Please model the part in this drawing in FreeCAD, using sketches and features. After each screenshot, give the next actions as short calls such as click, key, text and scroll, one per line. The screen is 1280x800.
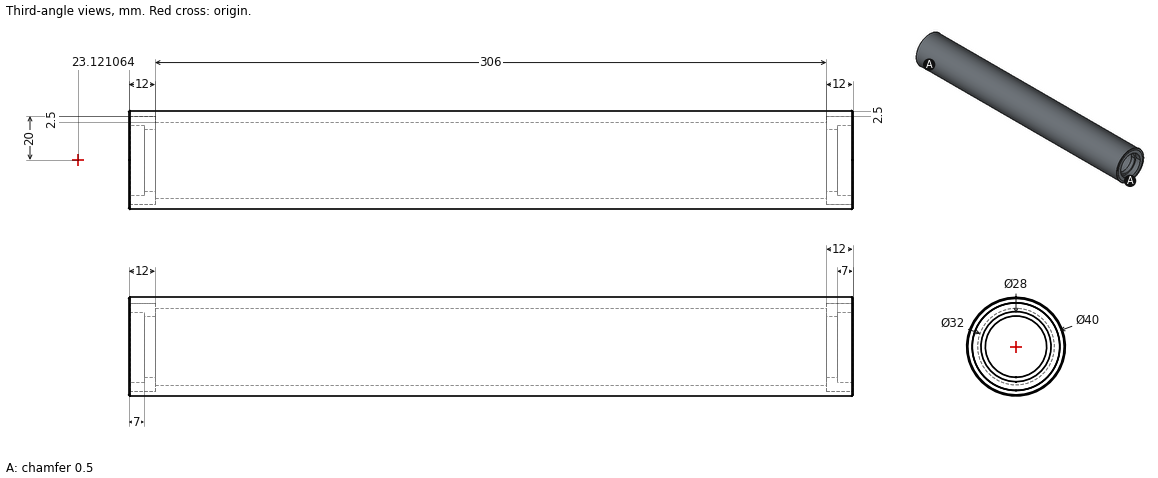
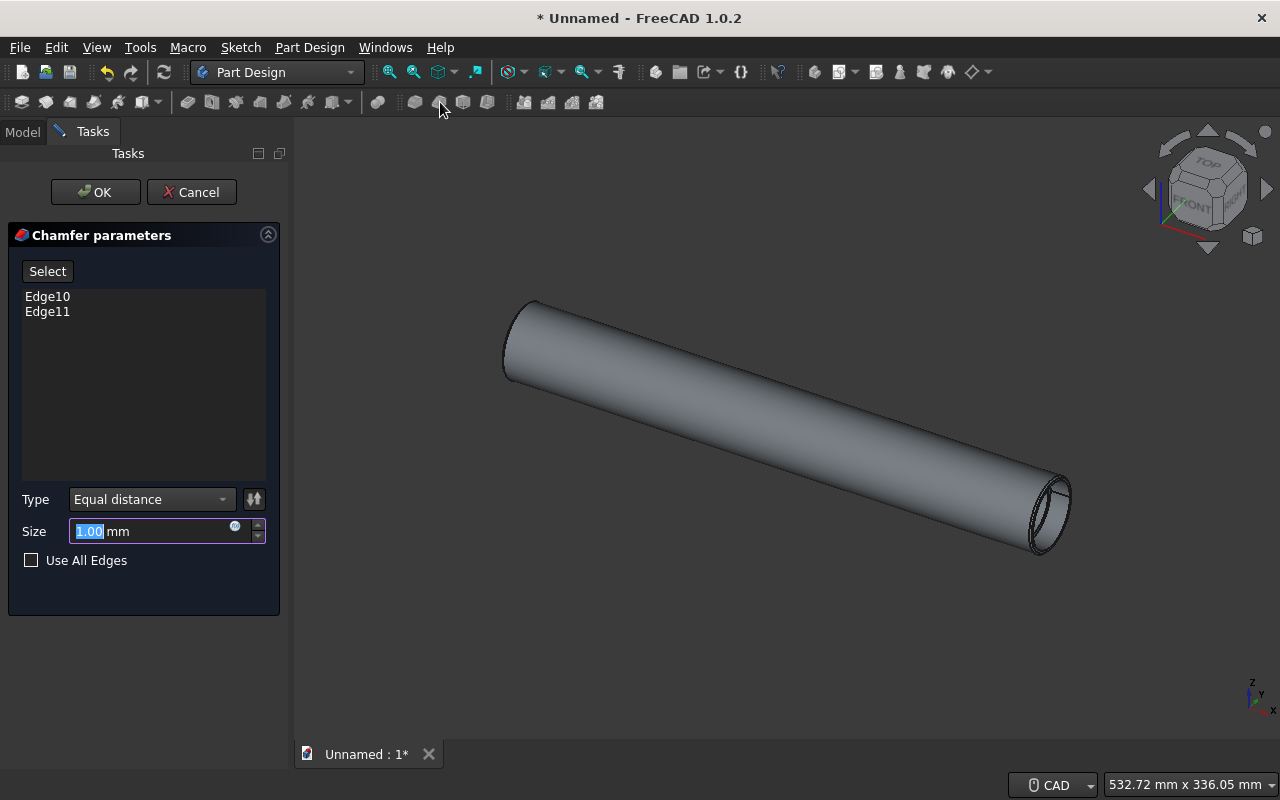
text(0.5)
key(Tab)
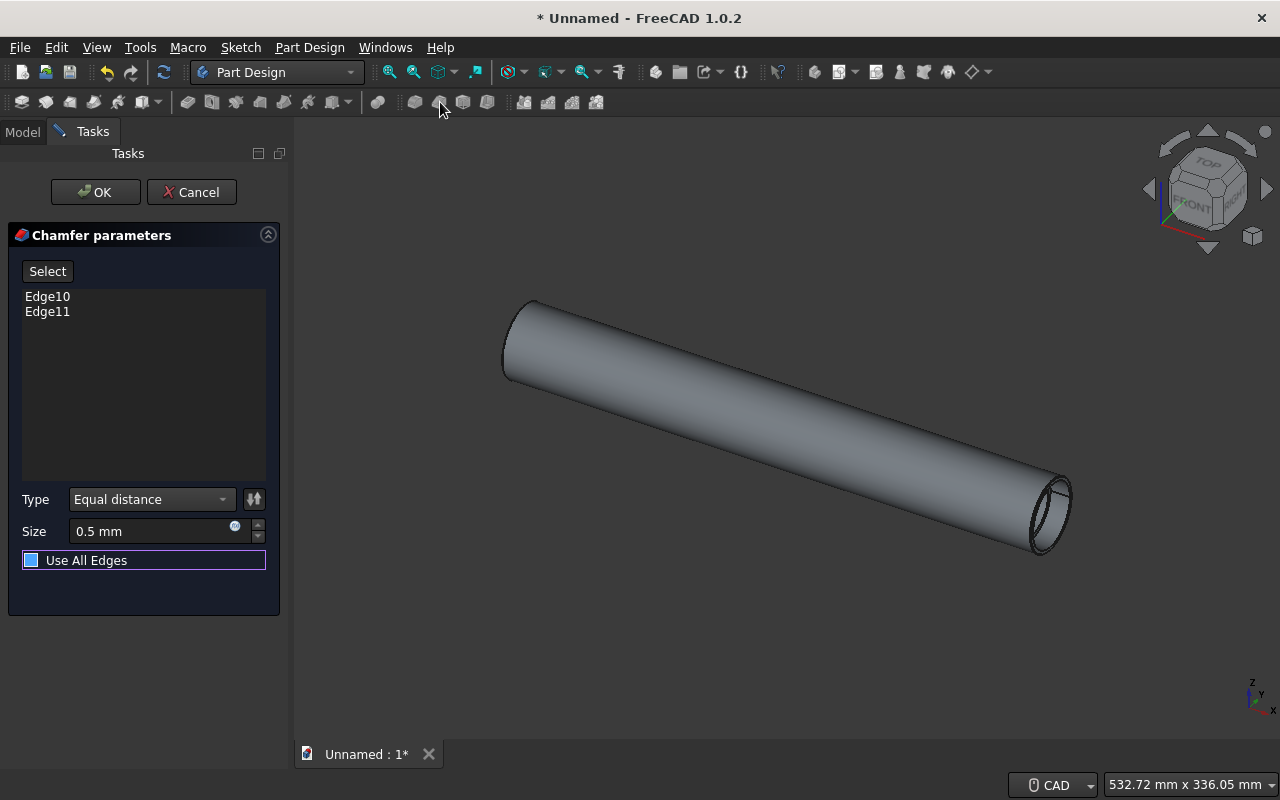
click(96, 192)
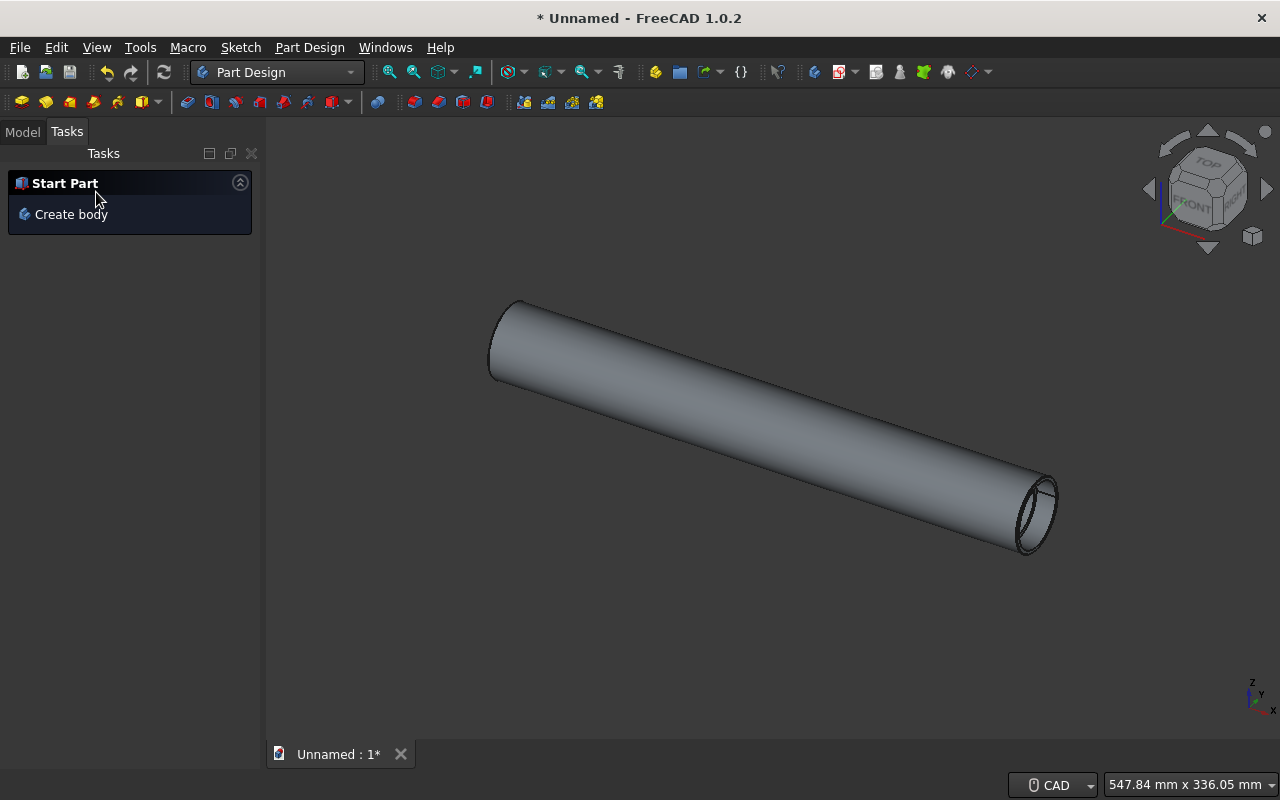
click(816, 72)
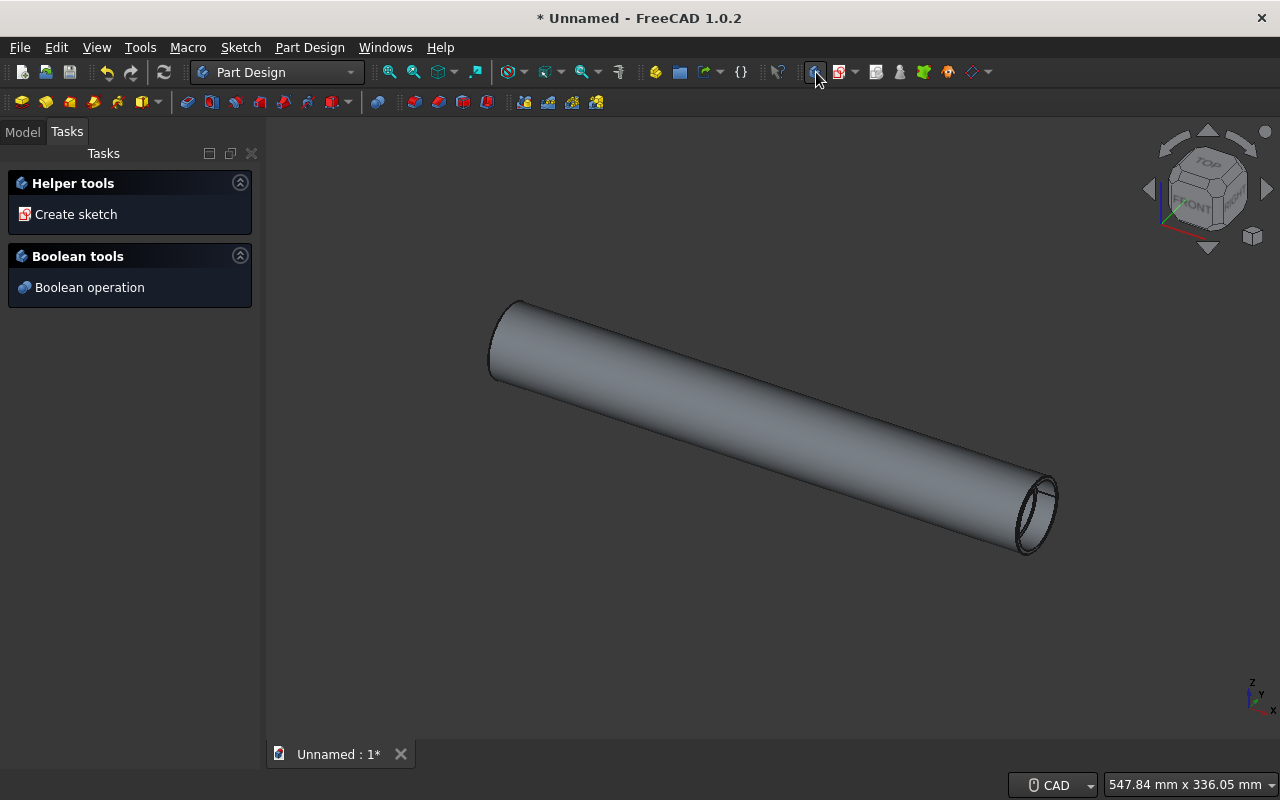
click(23, 131)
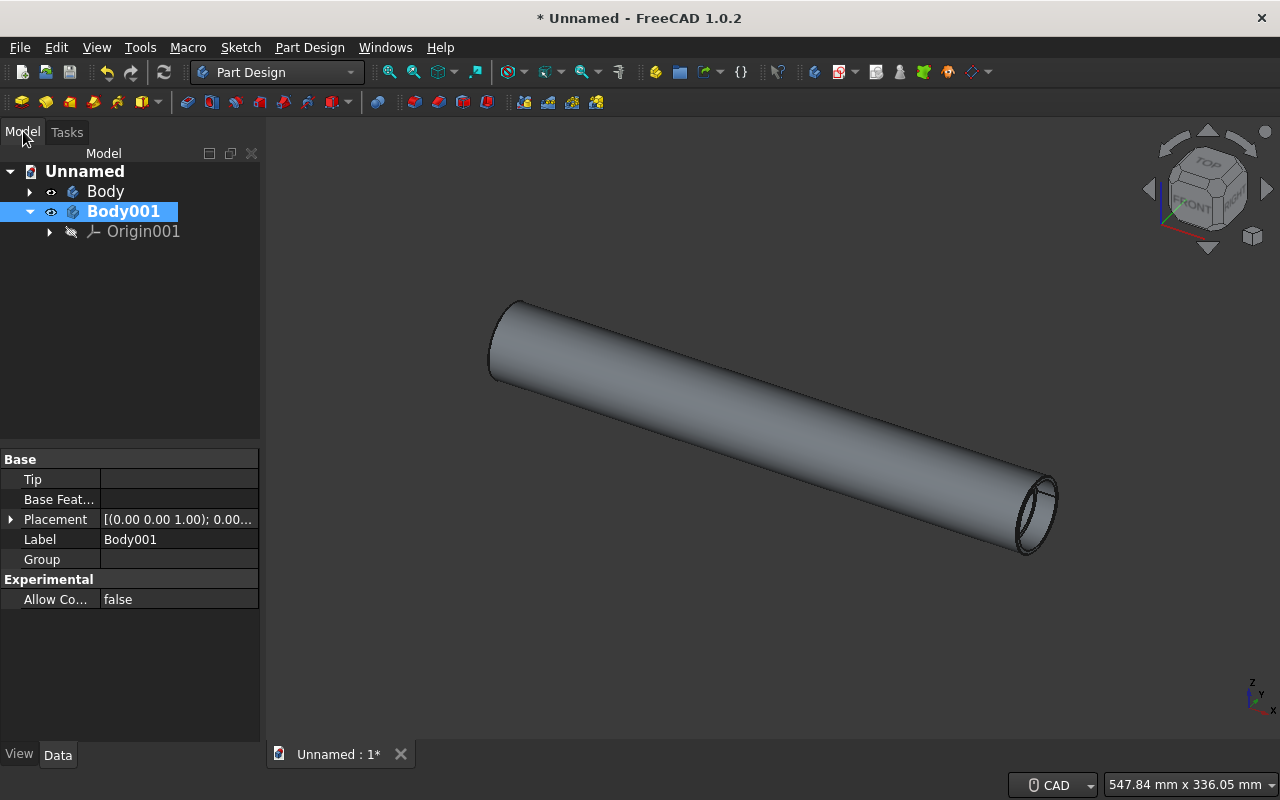
click(50, 232)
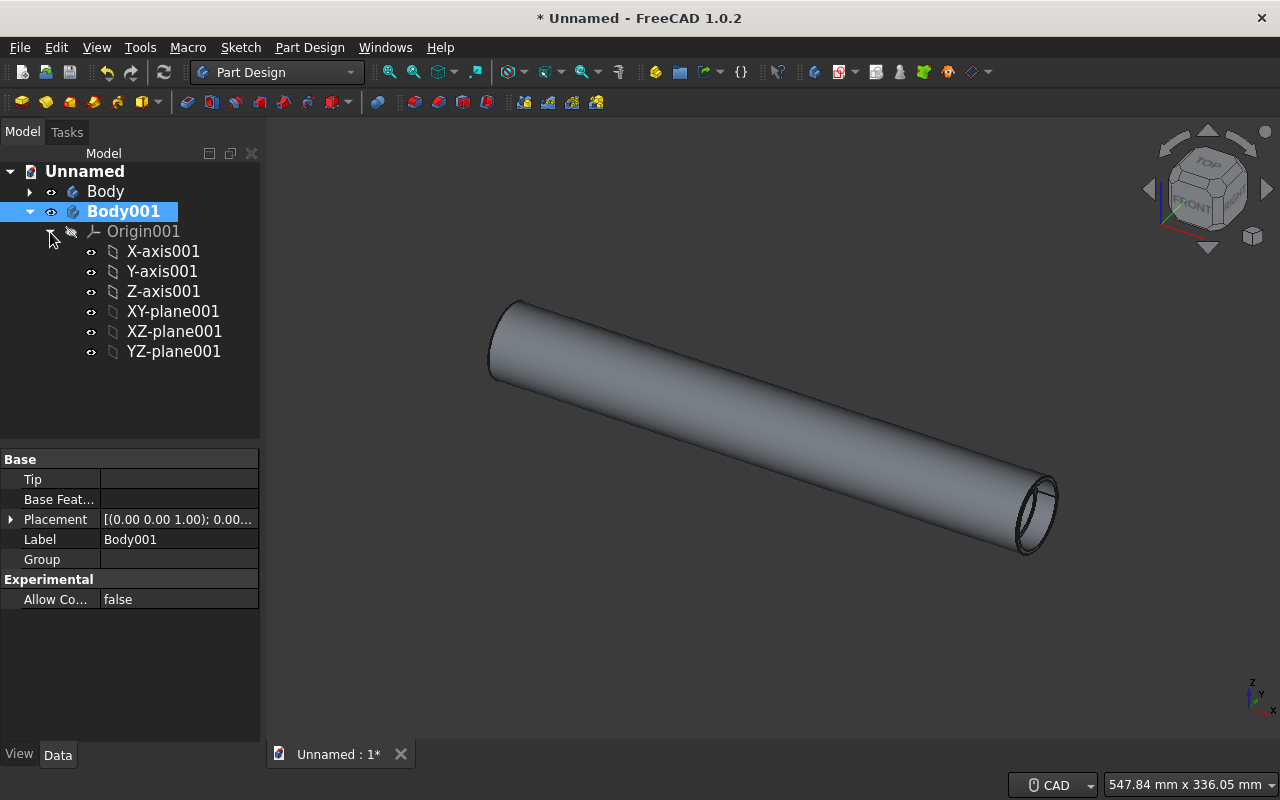
click(136, 352)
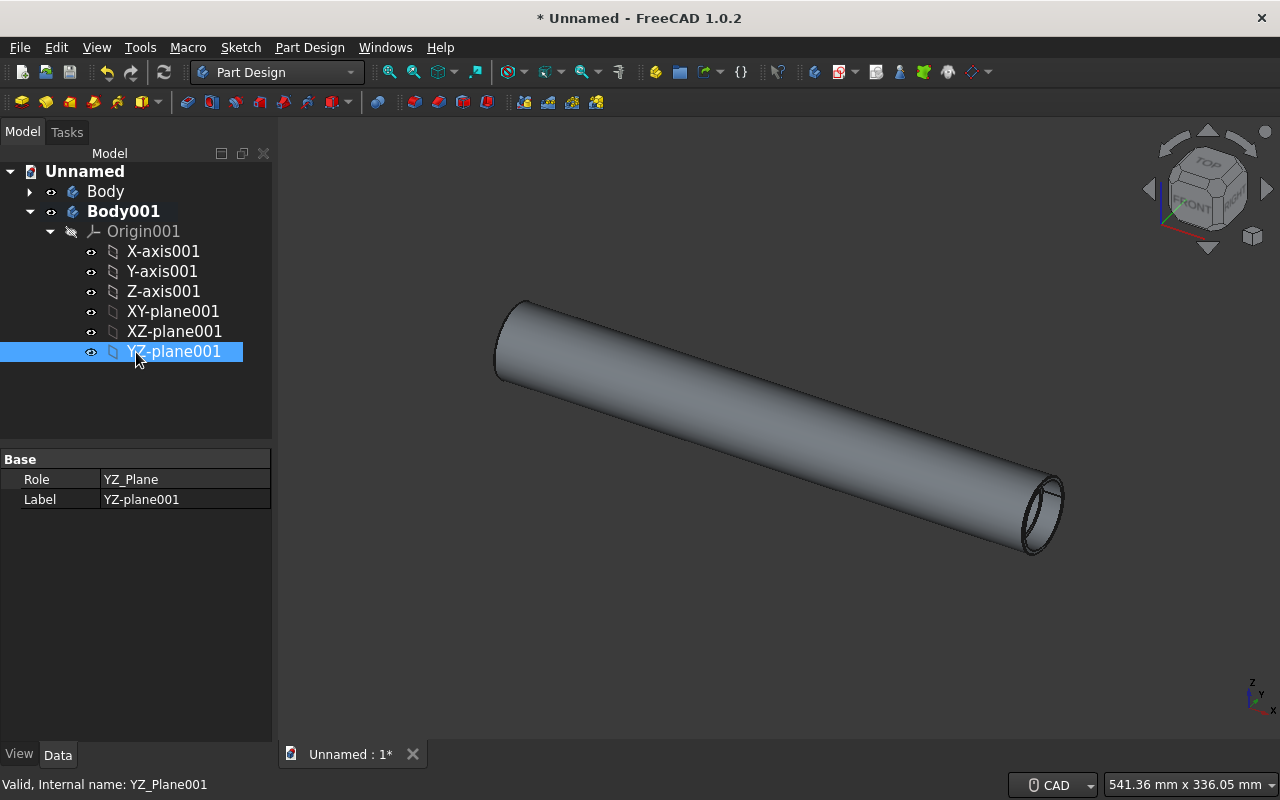
click(972, 72)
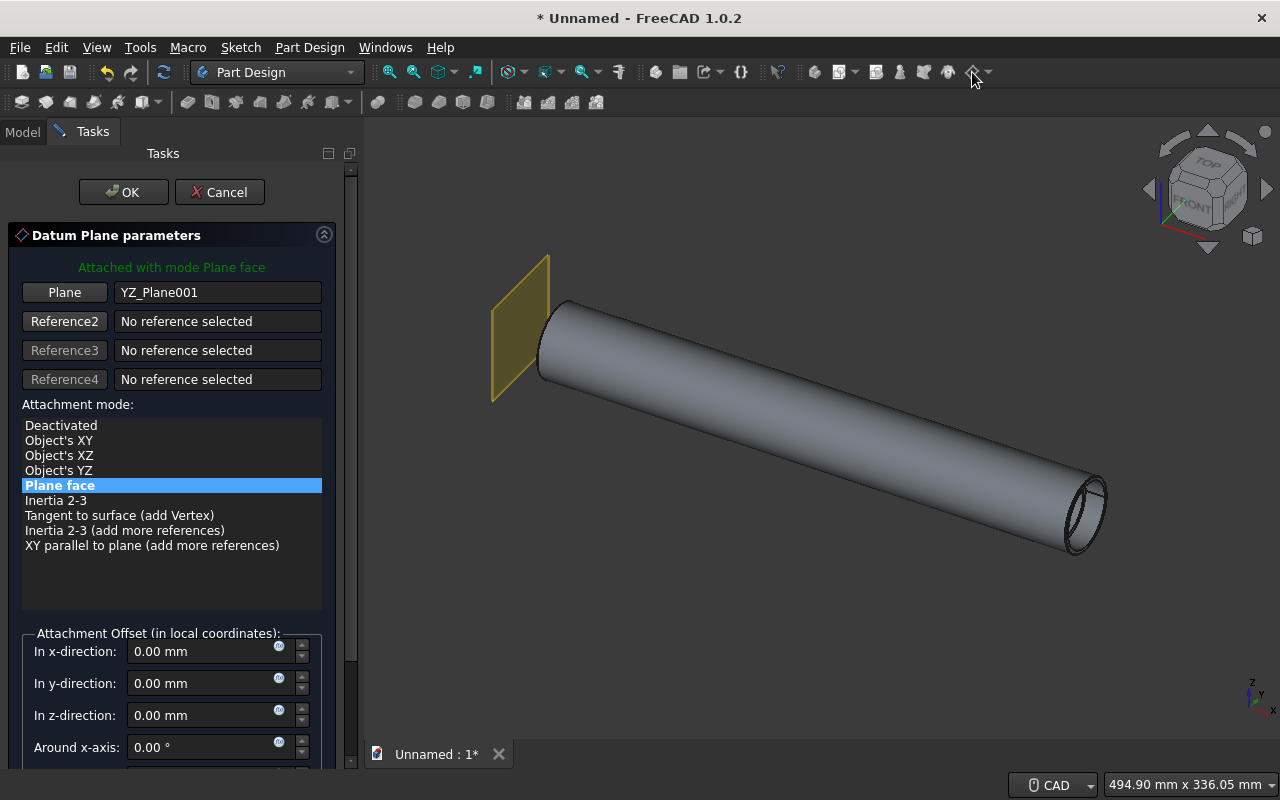
triple_click(210, 715)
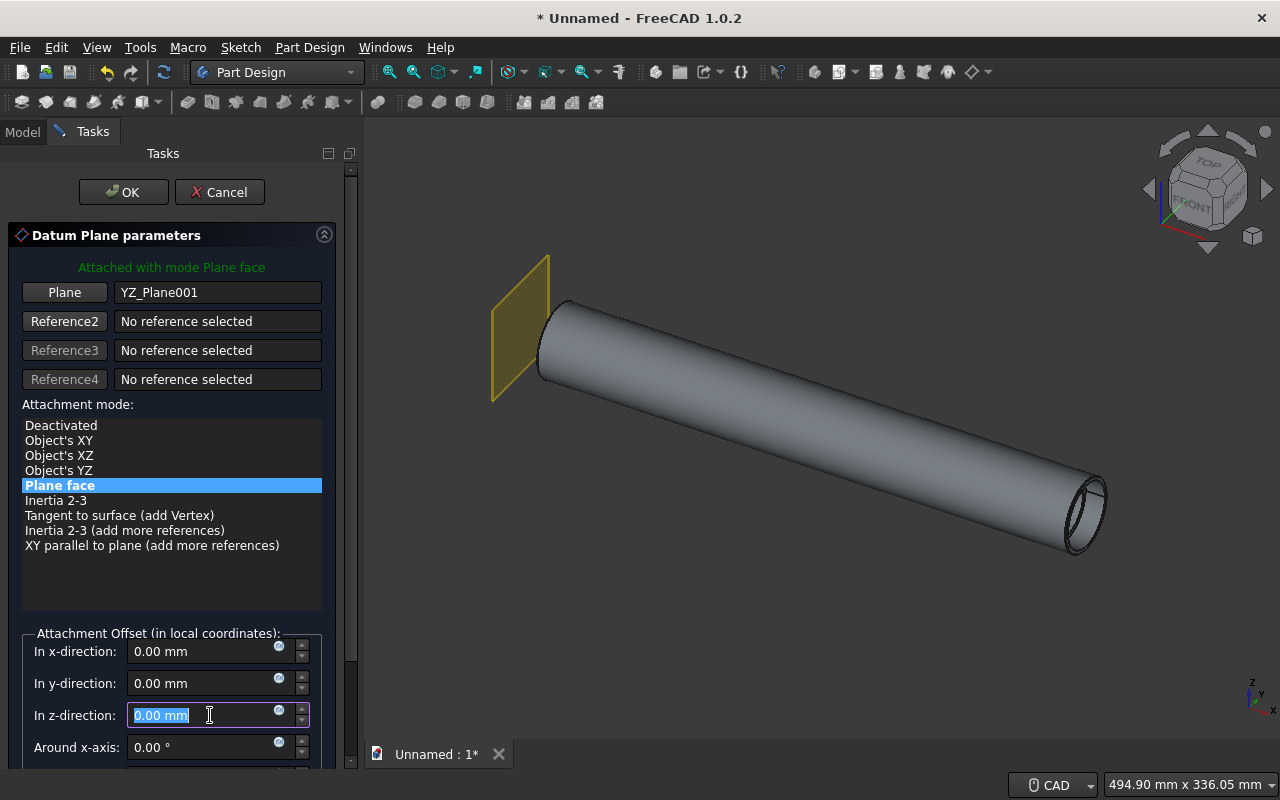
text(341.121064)
key(Tab)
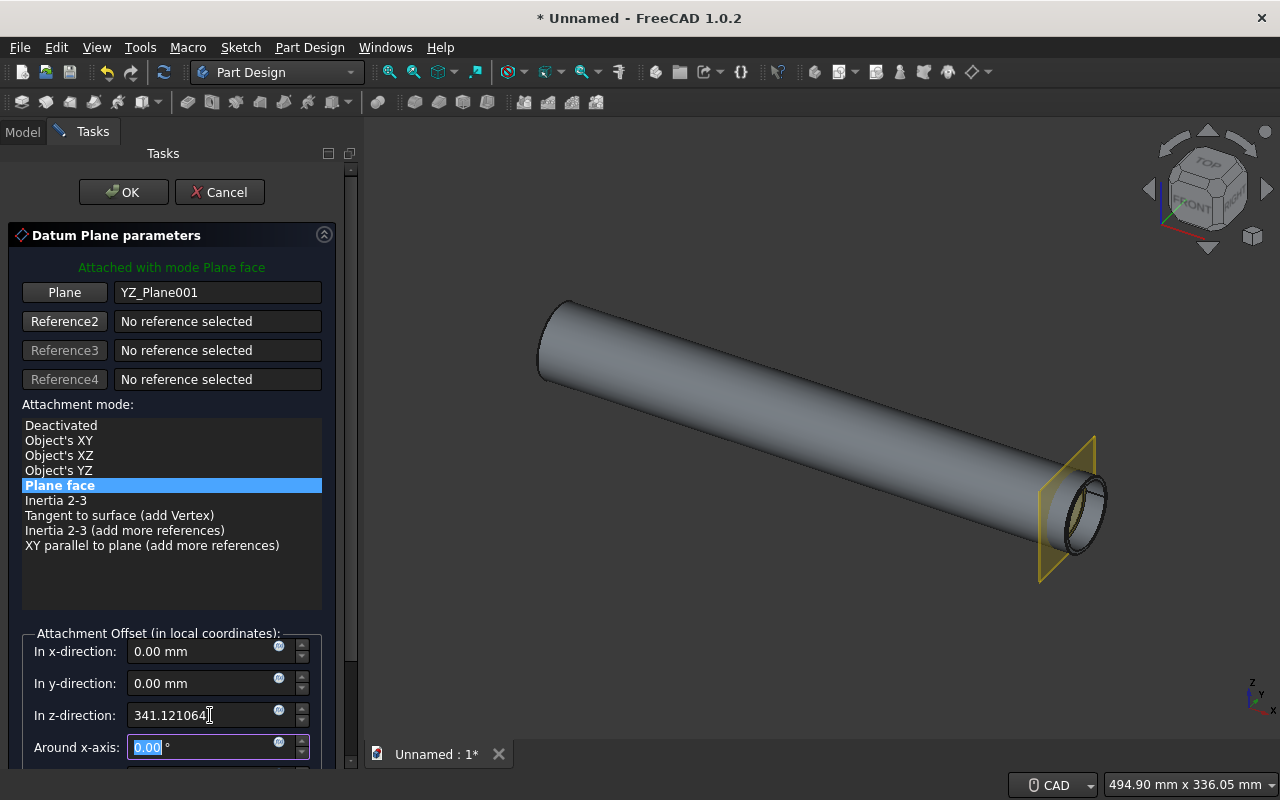
click(124, 192)